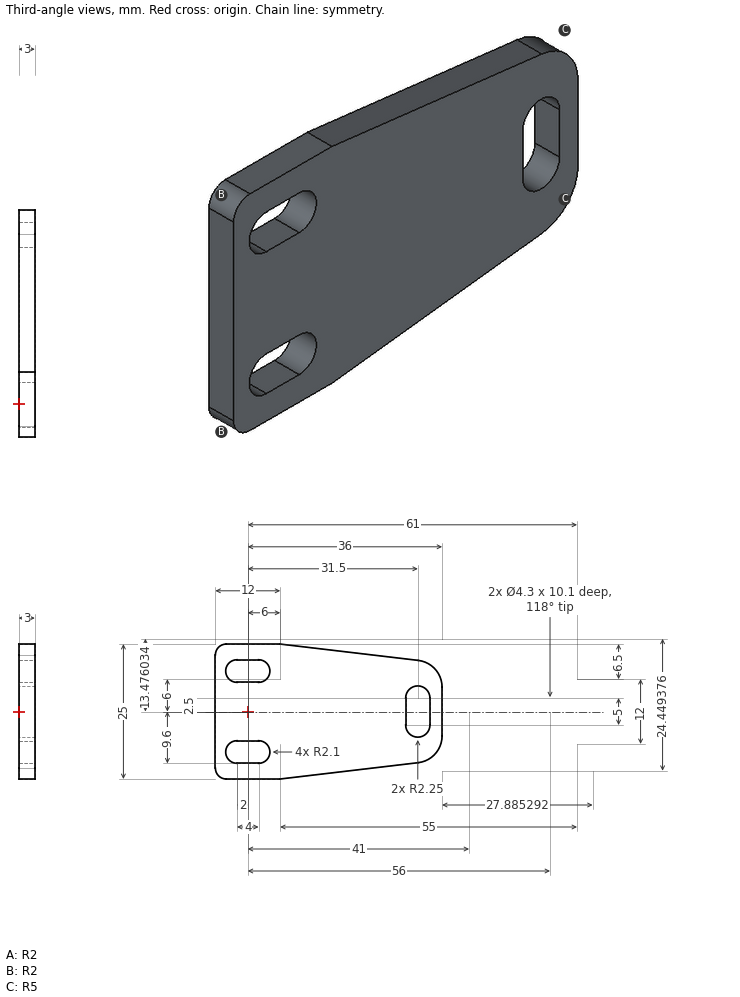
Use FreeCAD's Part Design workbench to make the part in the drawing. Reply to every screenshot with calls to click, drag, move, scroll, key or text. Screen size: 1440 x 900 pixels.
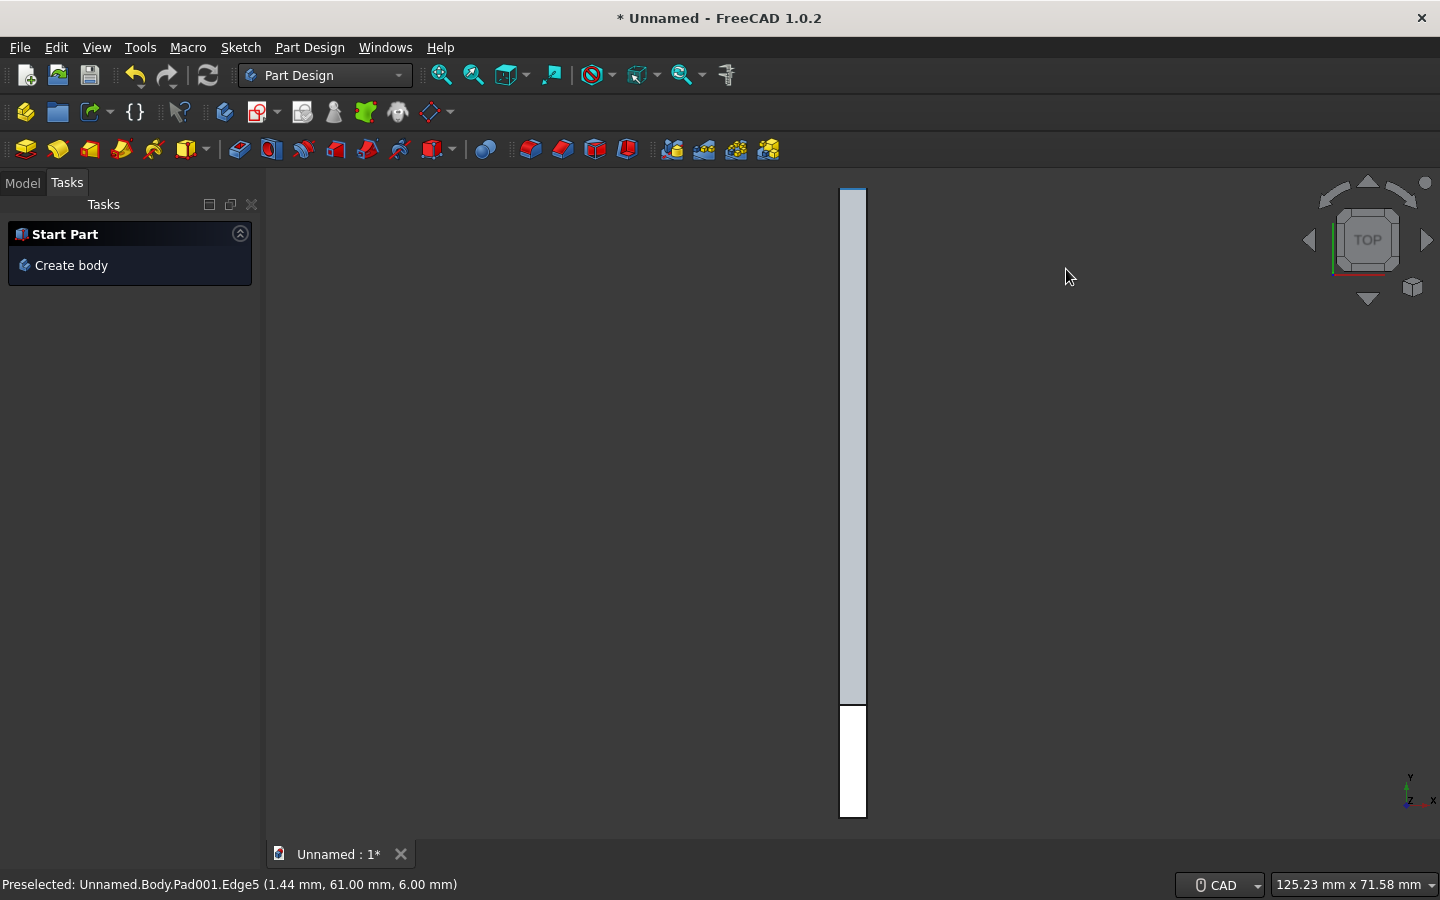
key(1)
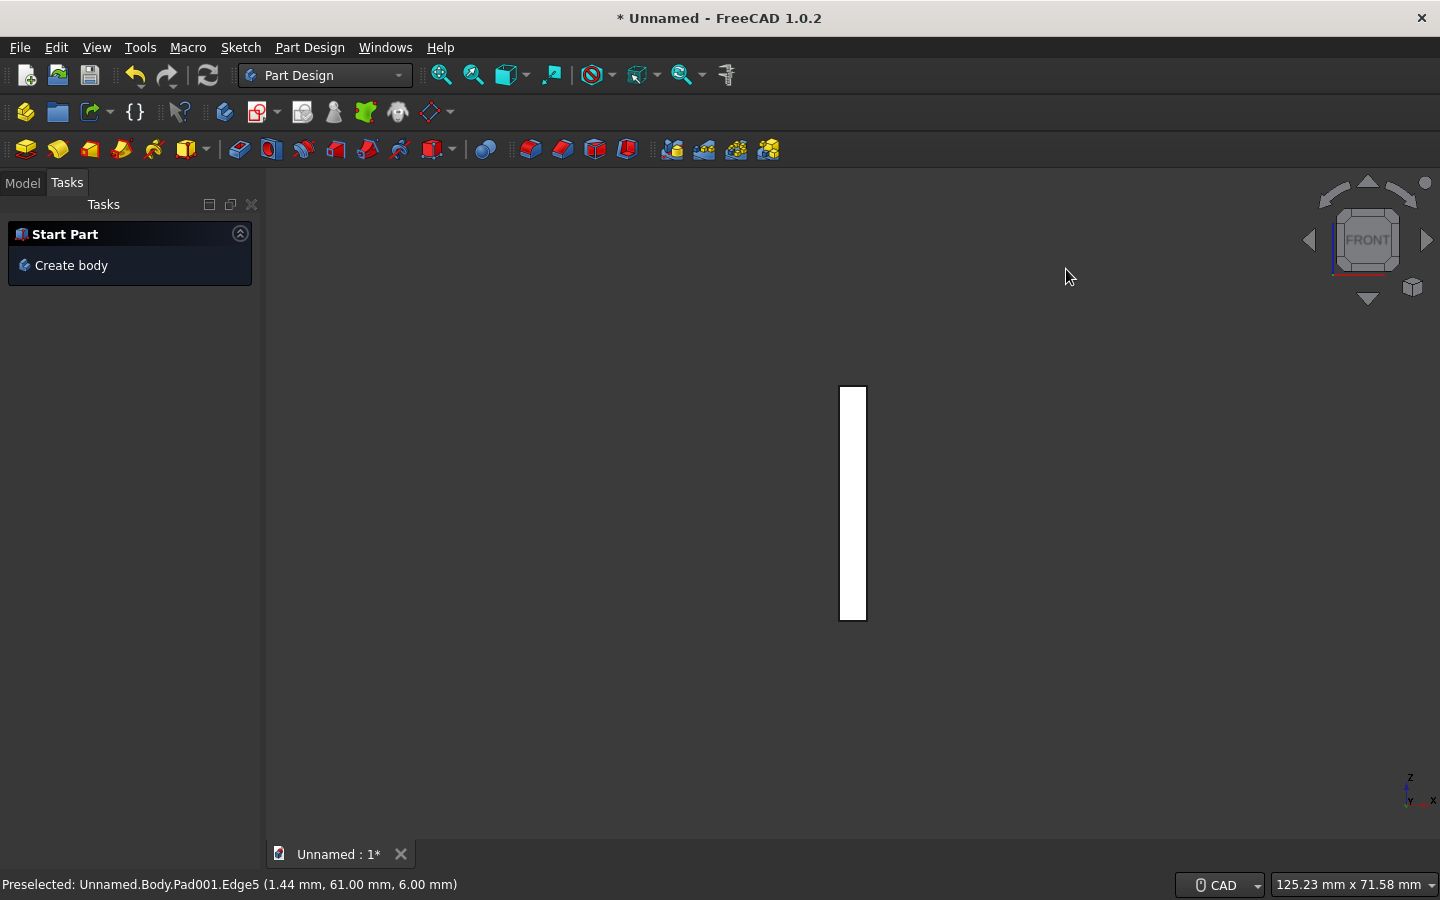
key(v)
key(f)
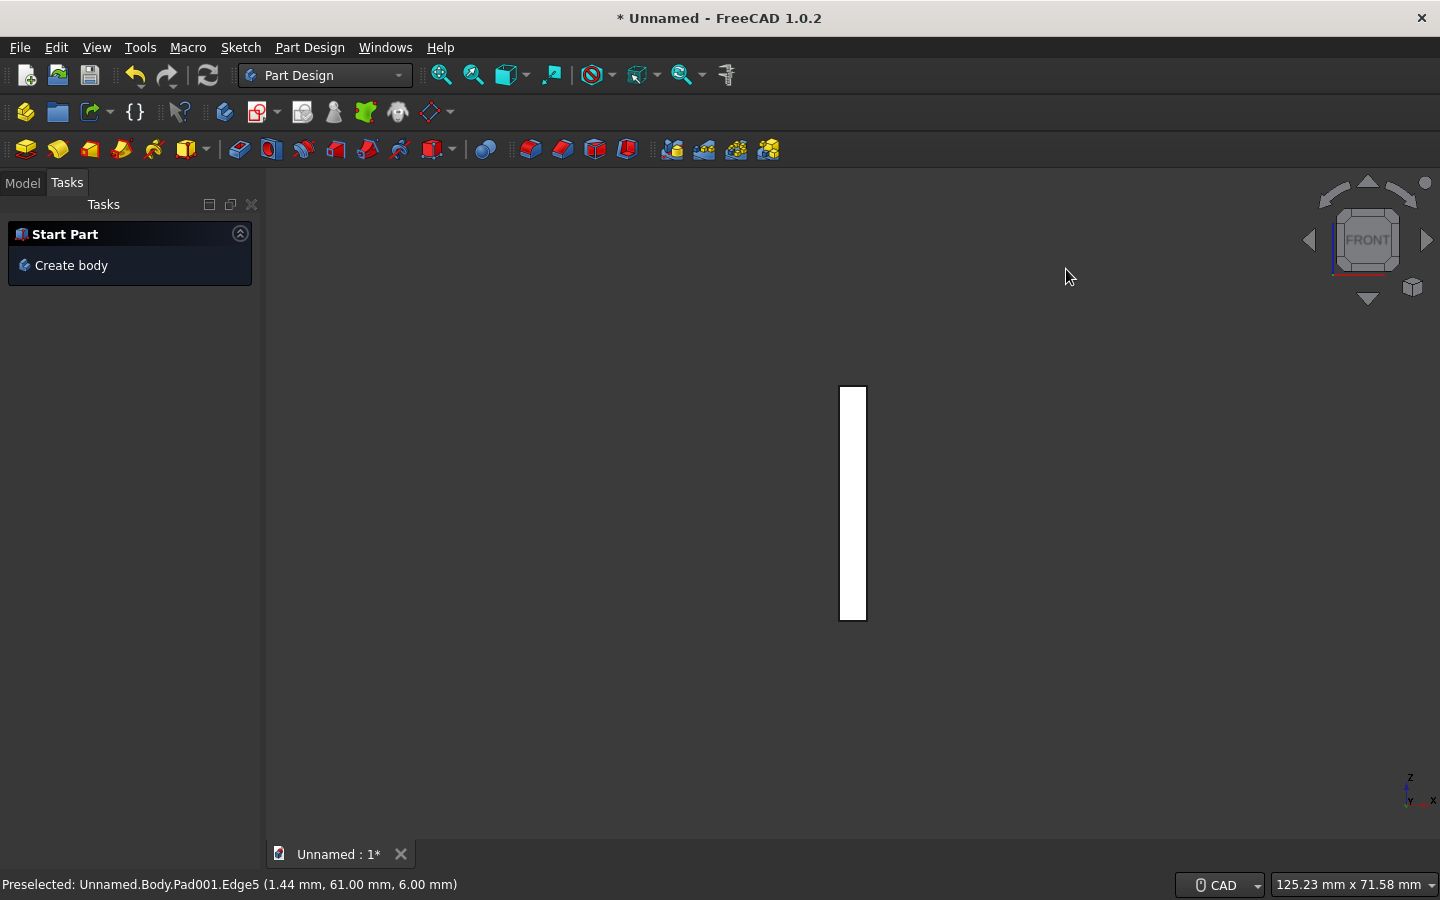
key(3)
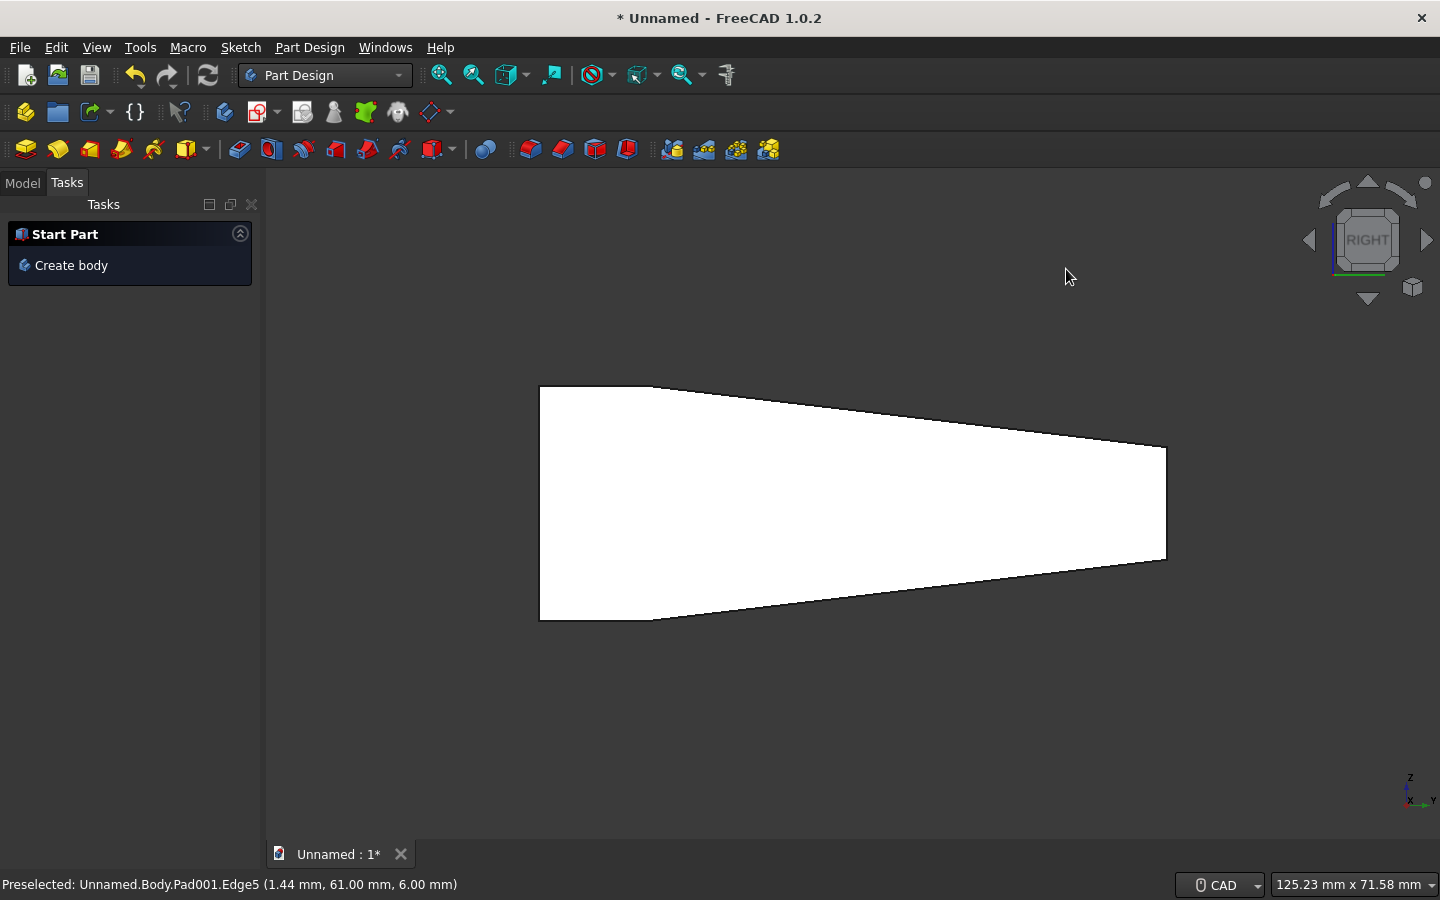
key(5)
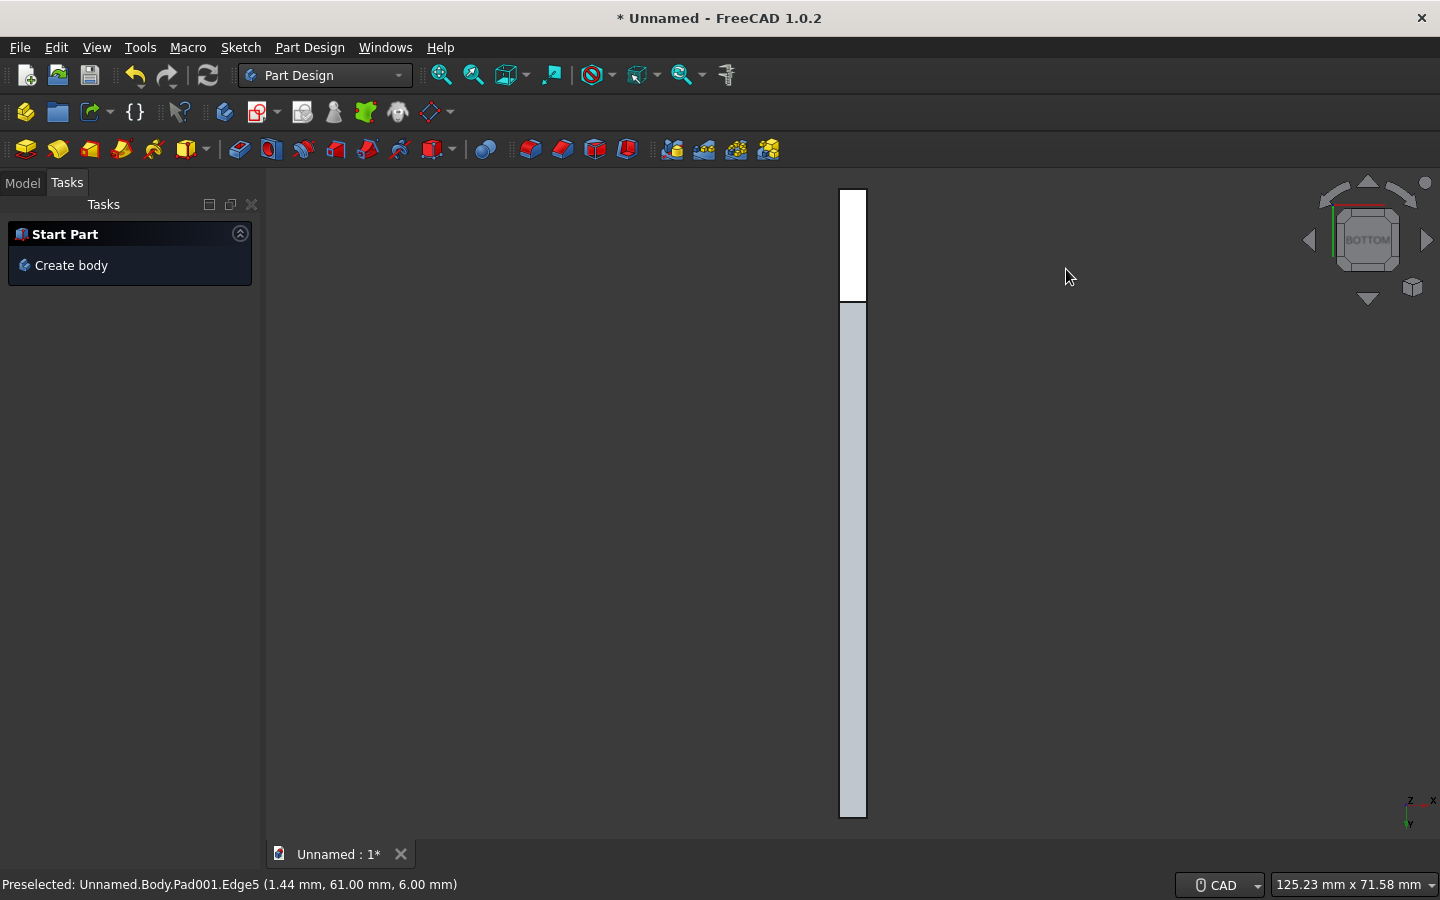
key(4)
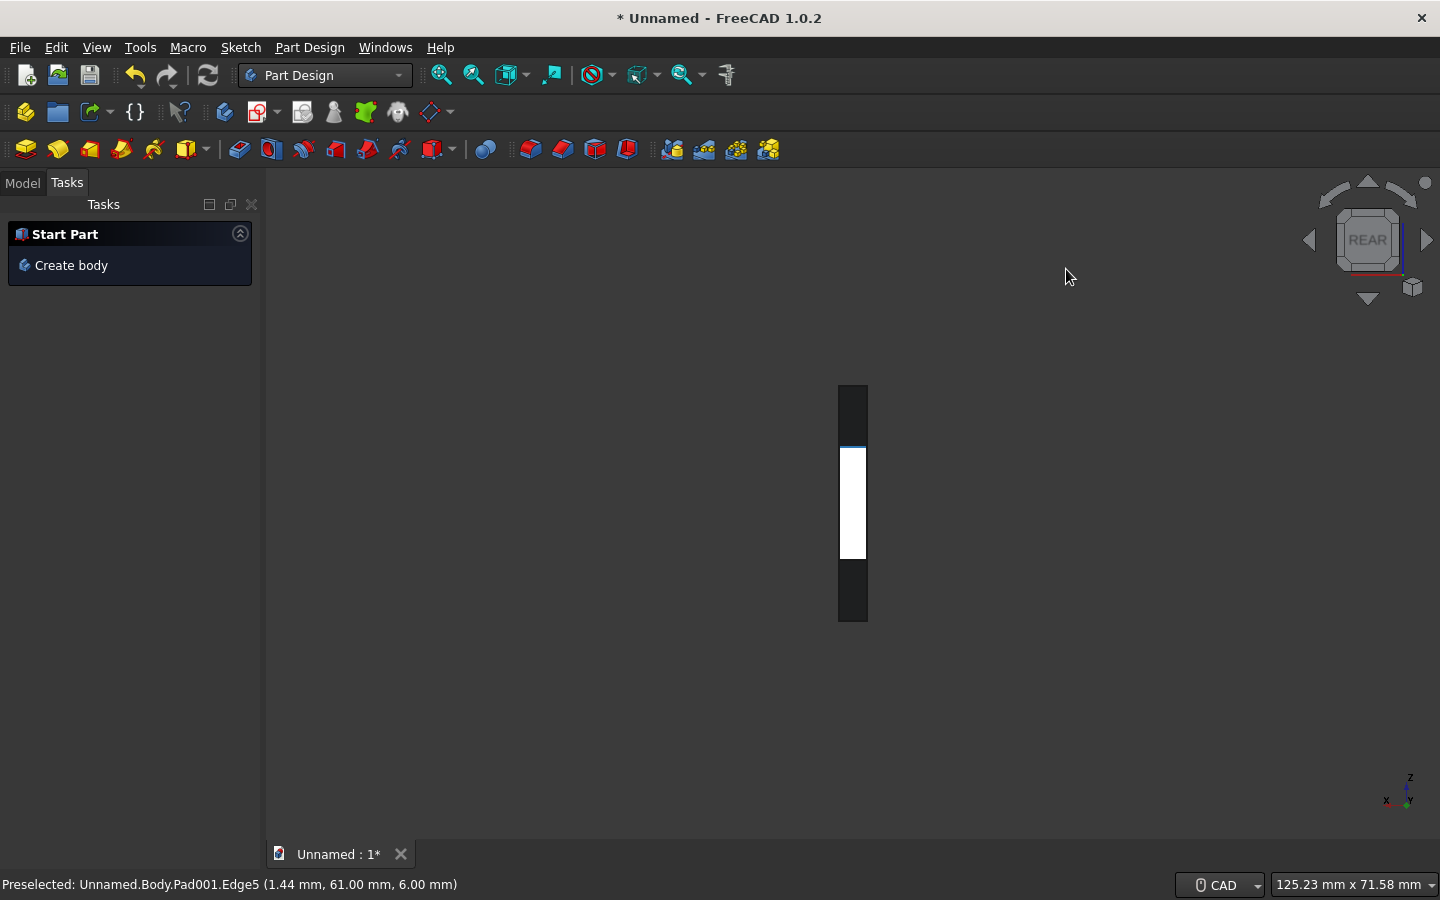
key(v)
key(f)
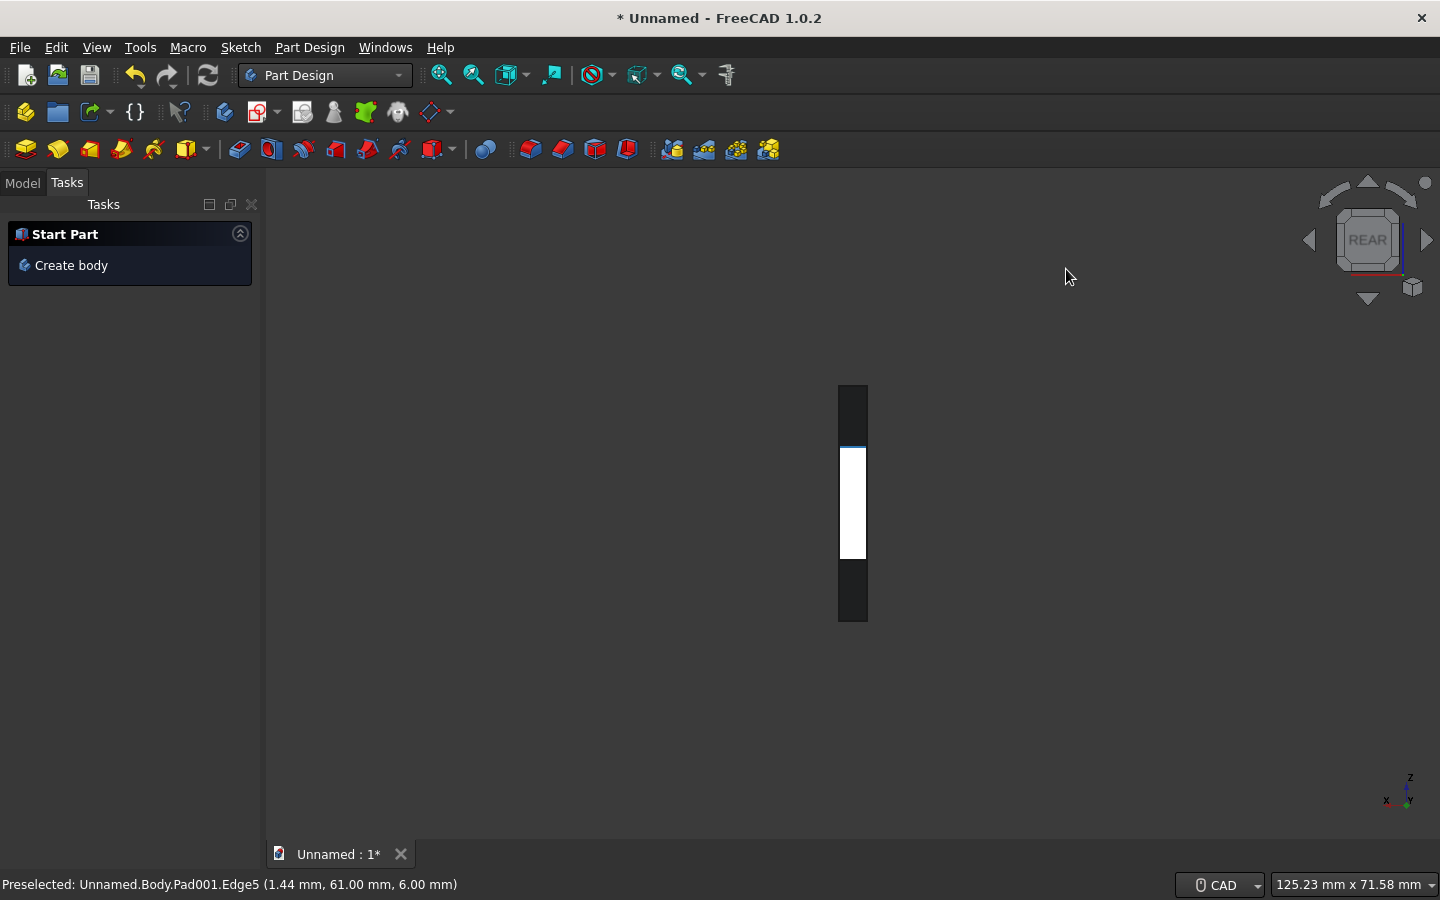
click(853, 446)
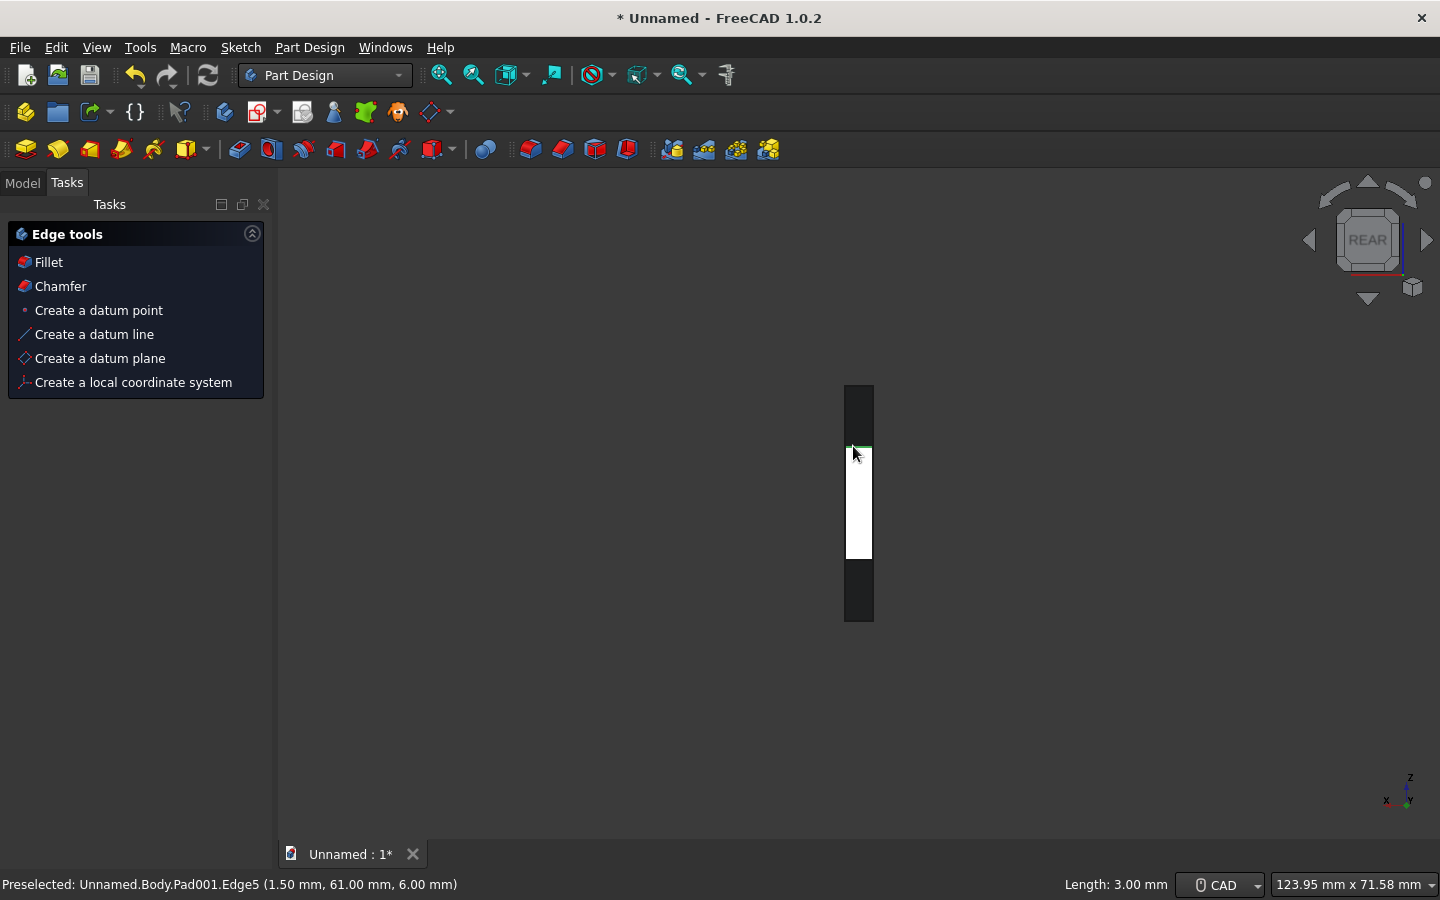
click(859, 559, ctrl)